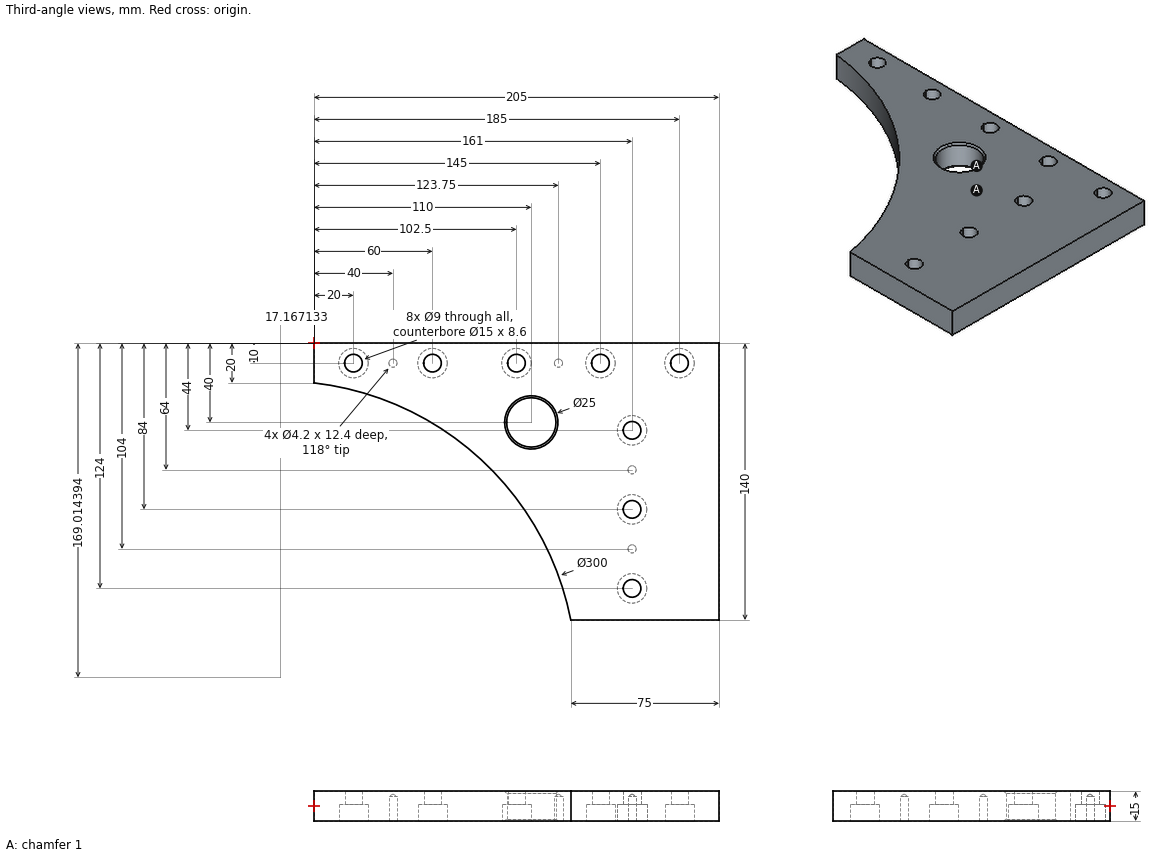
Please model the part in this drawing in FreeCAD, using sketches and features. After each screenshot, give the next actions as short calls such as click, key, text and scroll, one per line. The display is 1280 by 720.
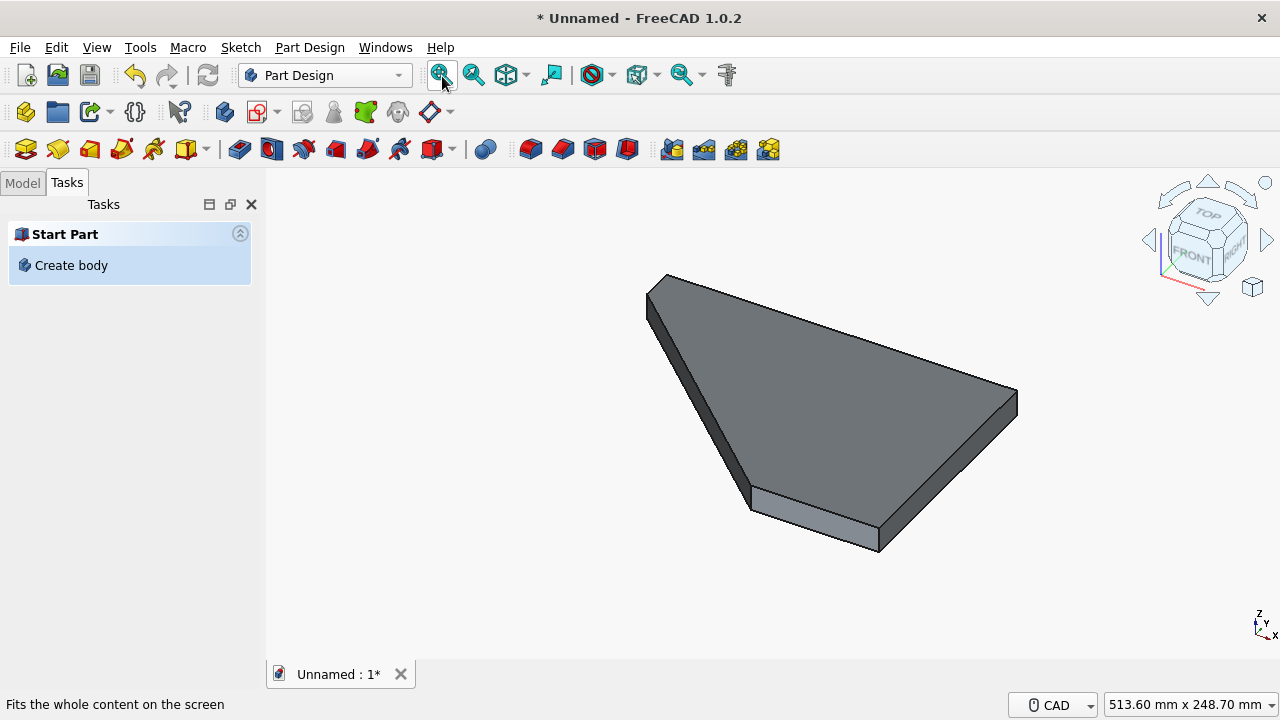
key(5)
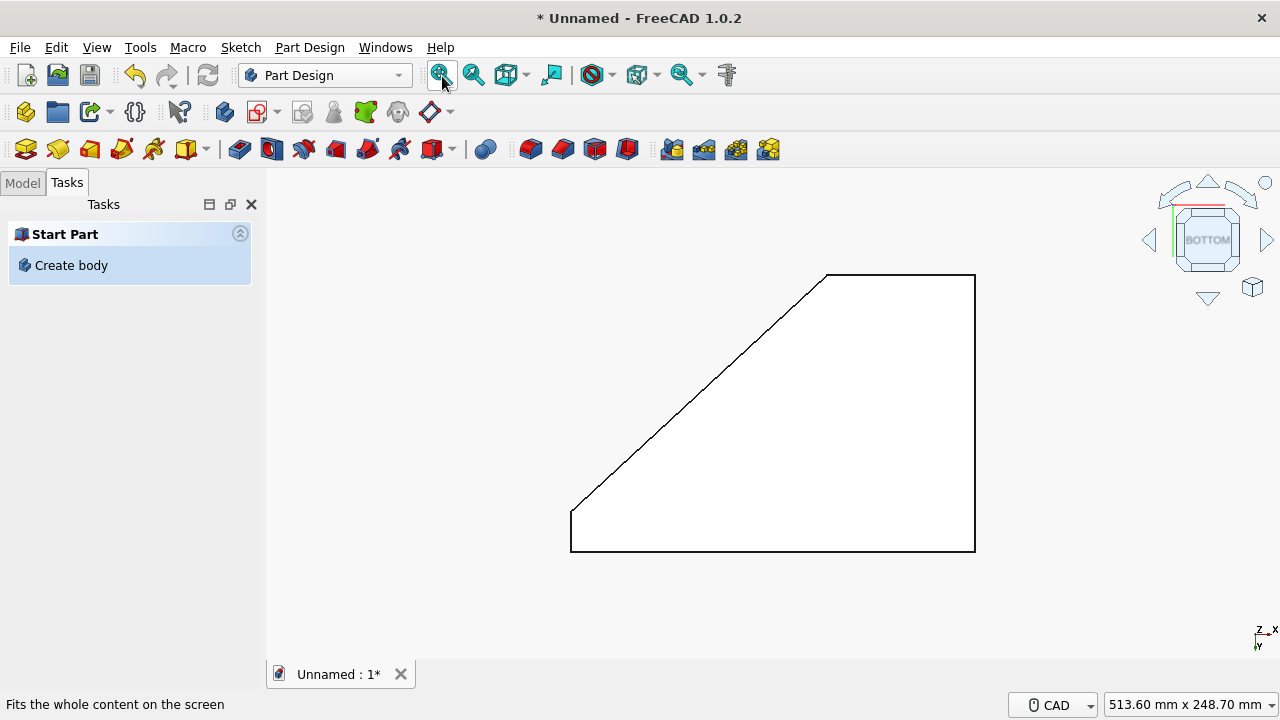
click(831, 412)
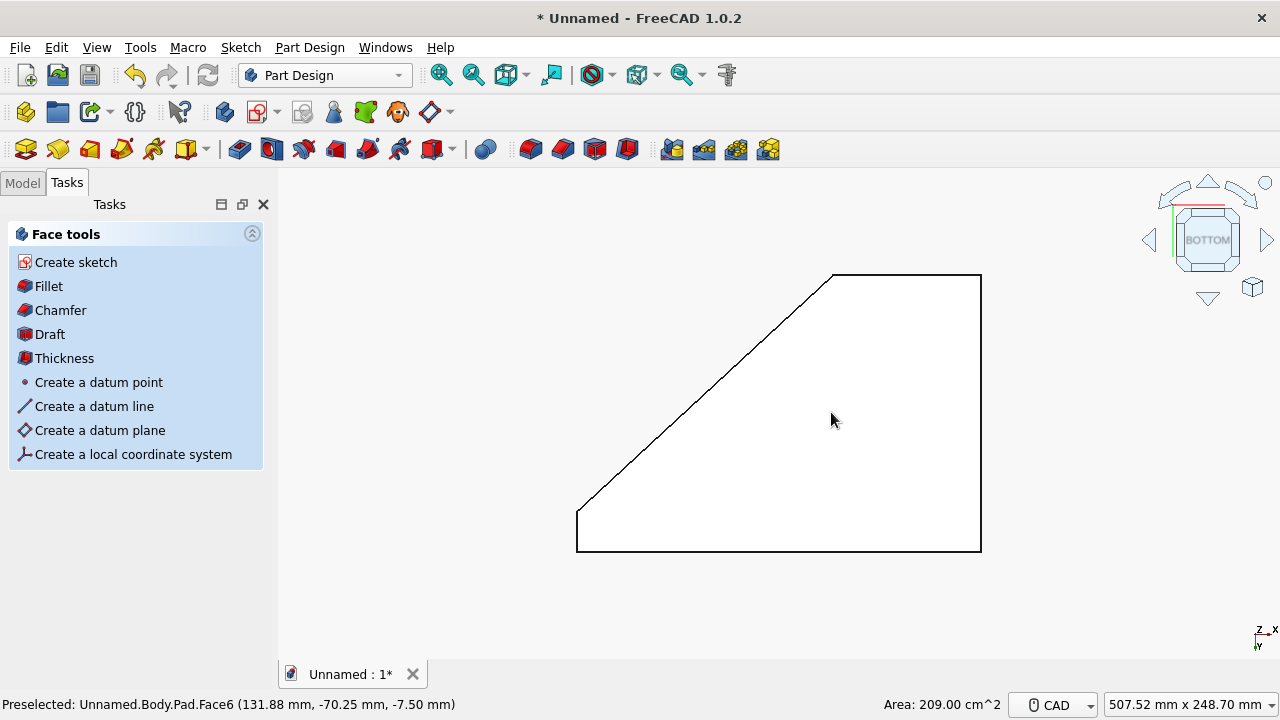
click(258, 112)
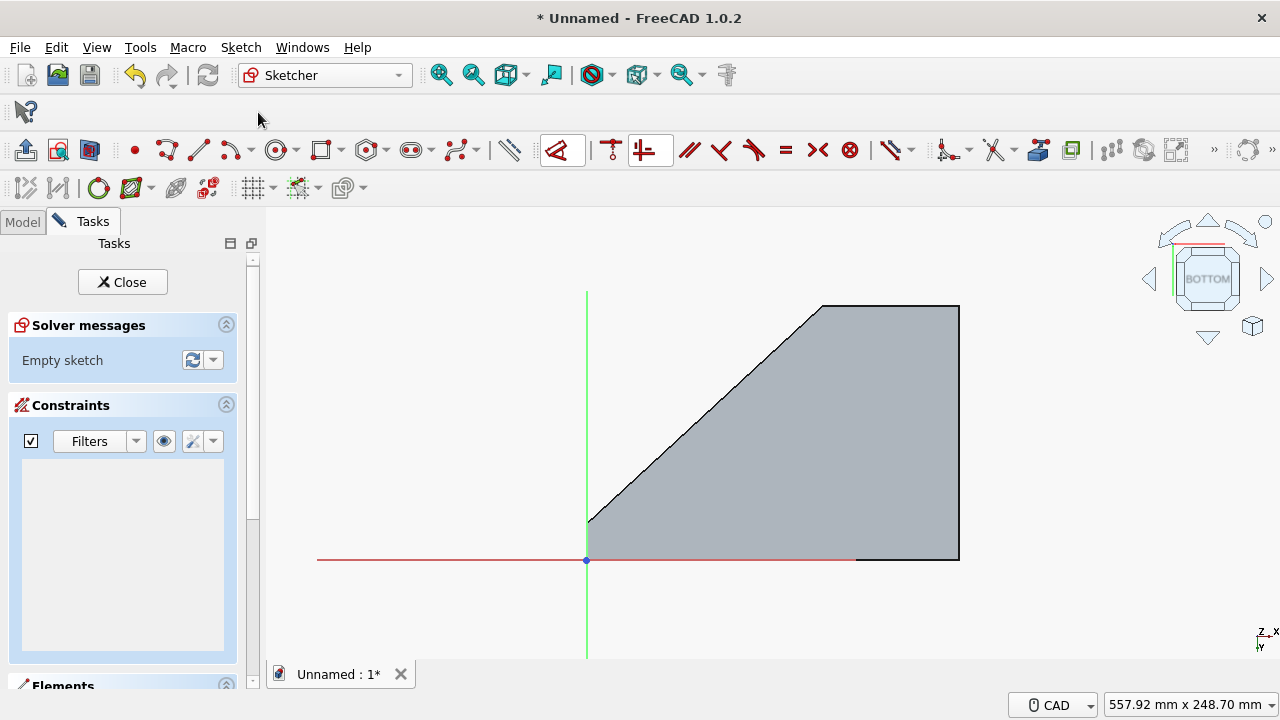
click(276, 150)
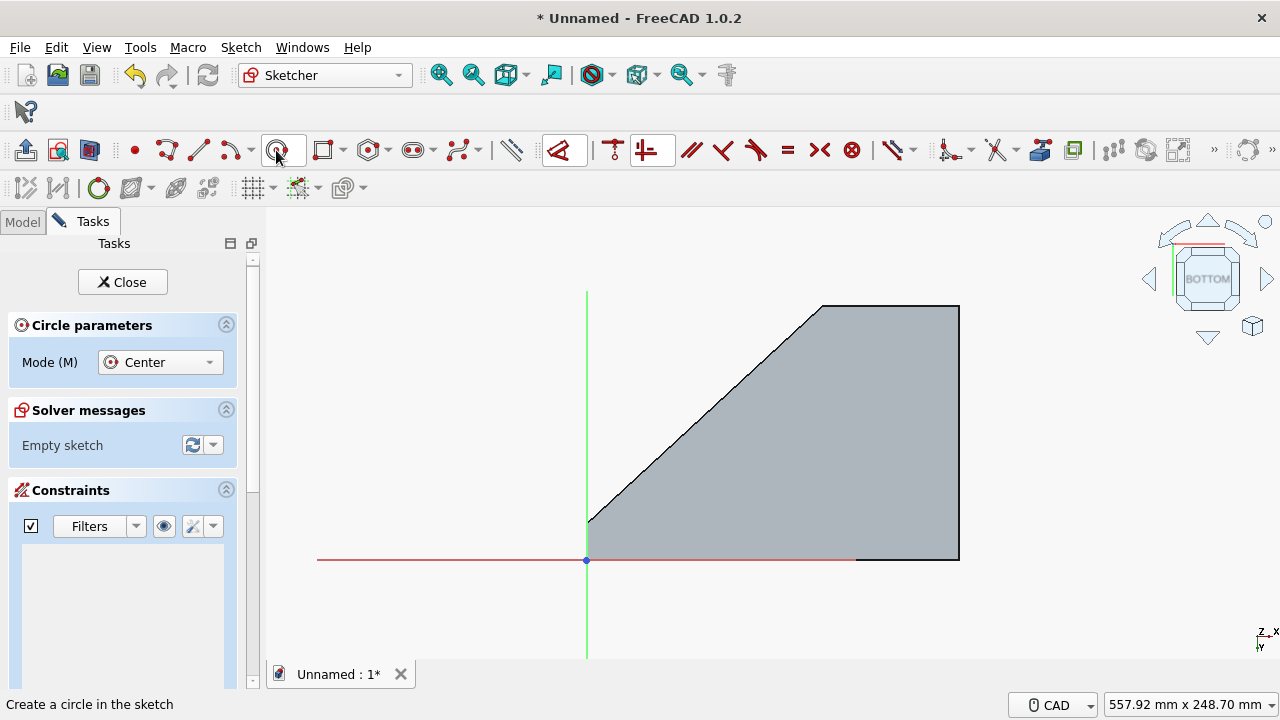
scroll(623, 542, up, 6)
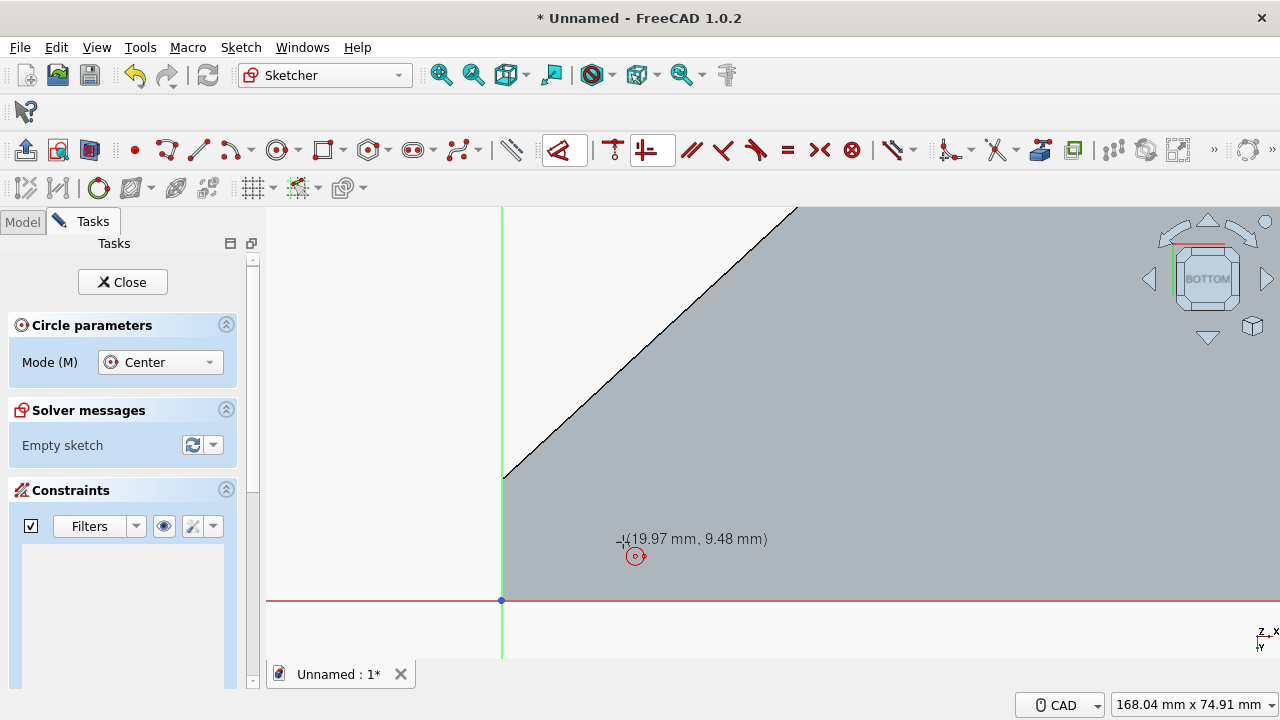
click(622, 540)
click(642, 521)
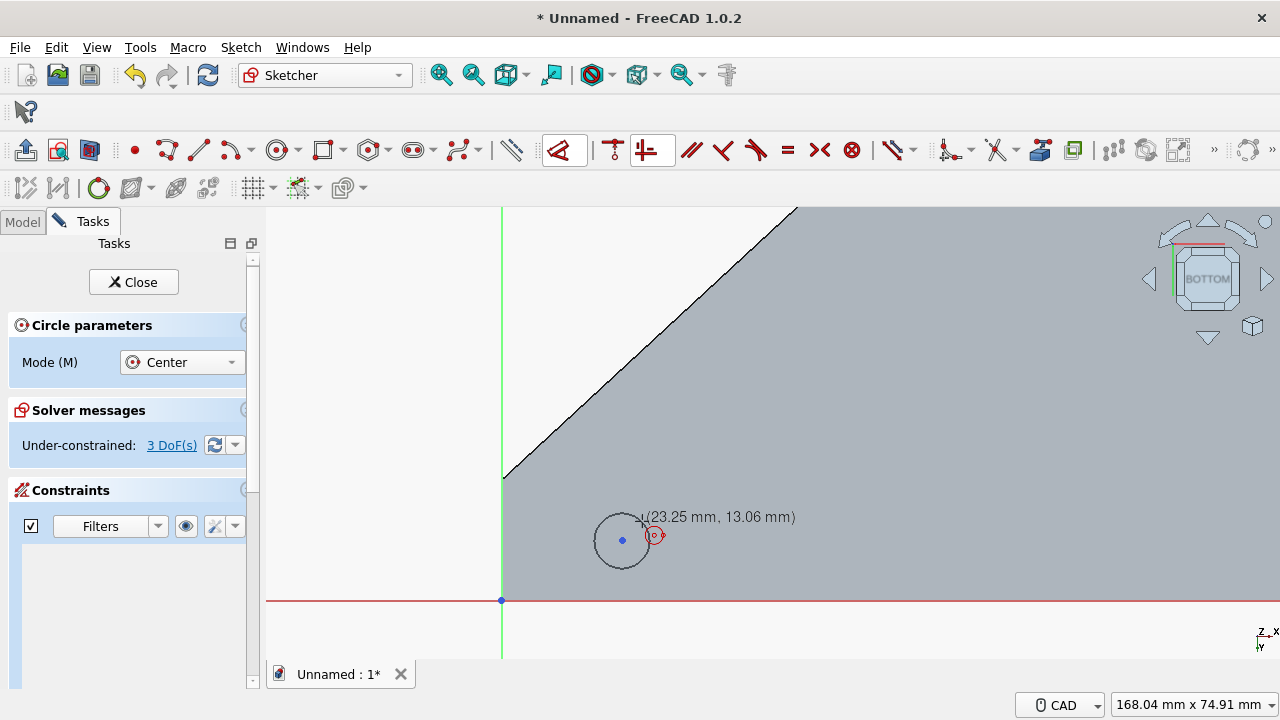
click(864, 540)
click(883, 521)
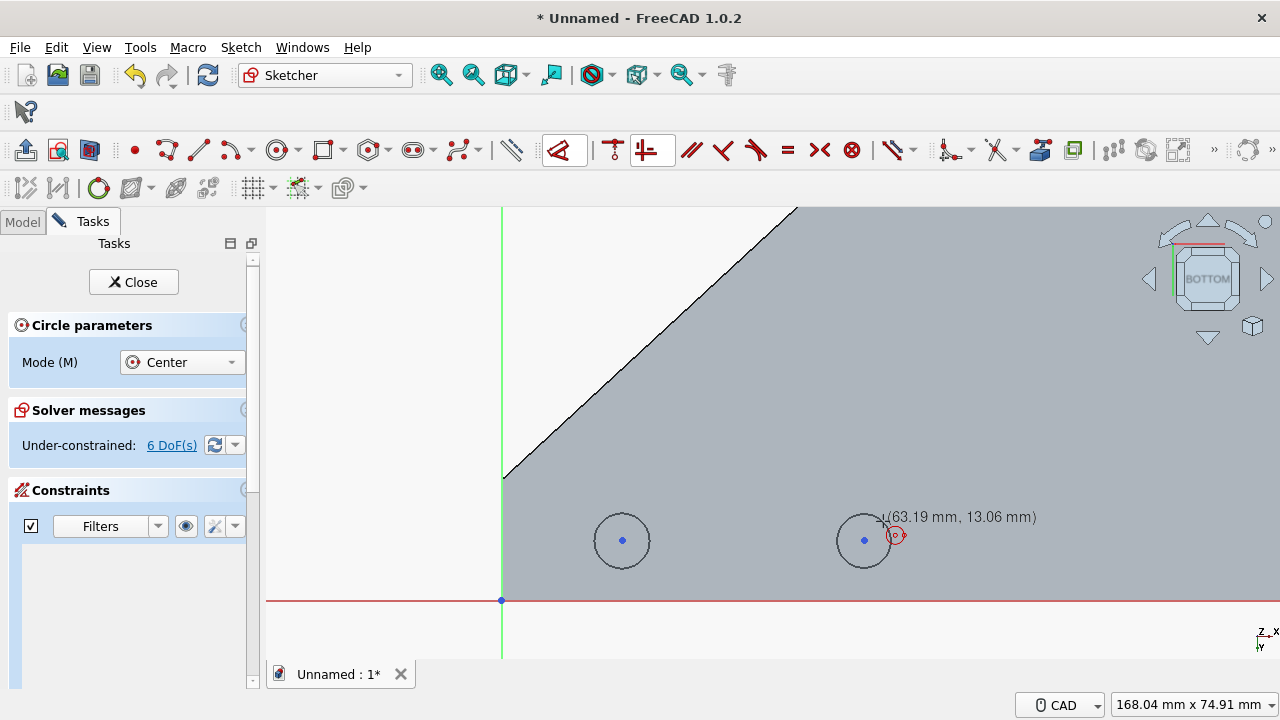
scroll(490, 561, down, 5)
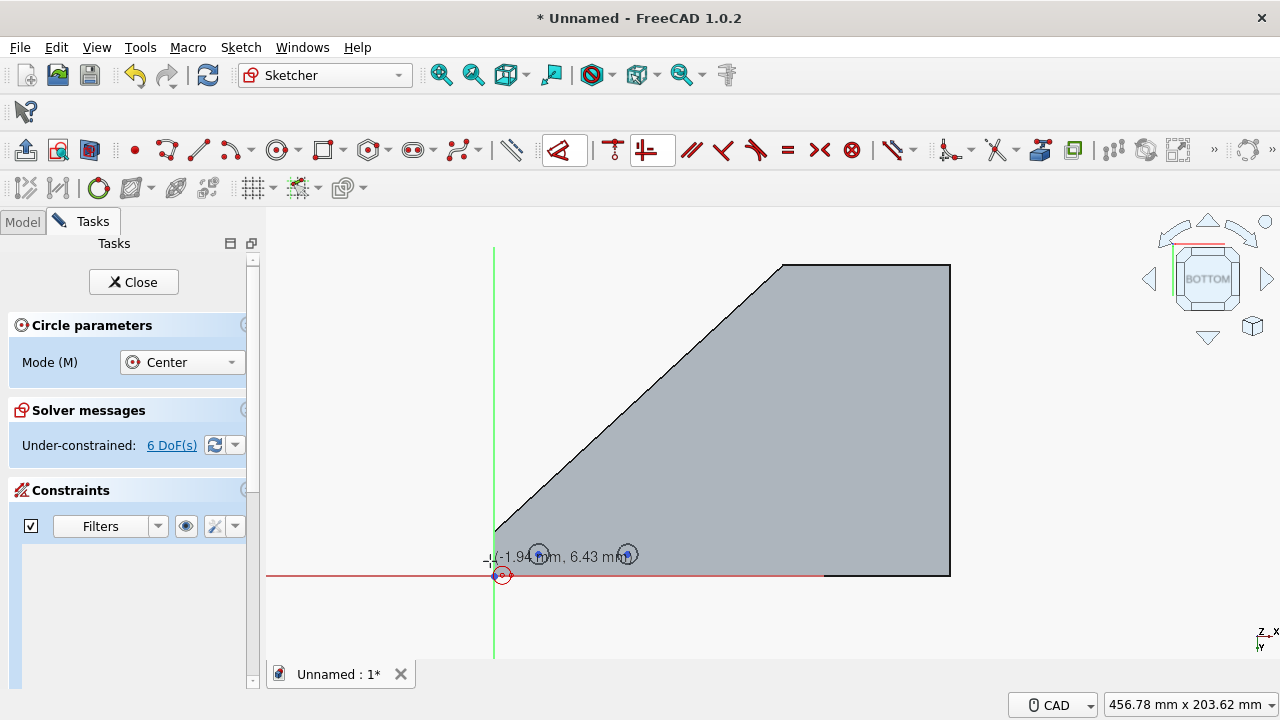
scroll(722, 554, up, 5)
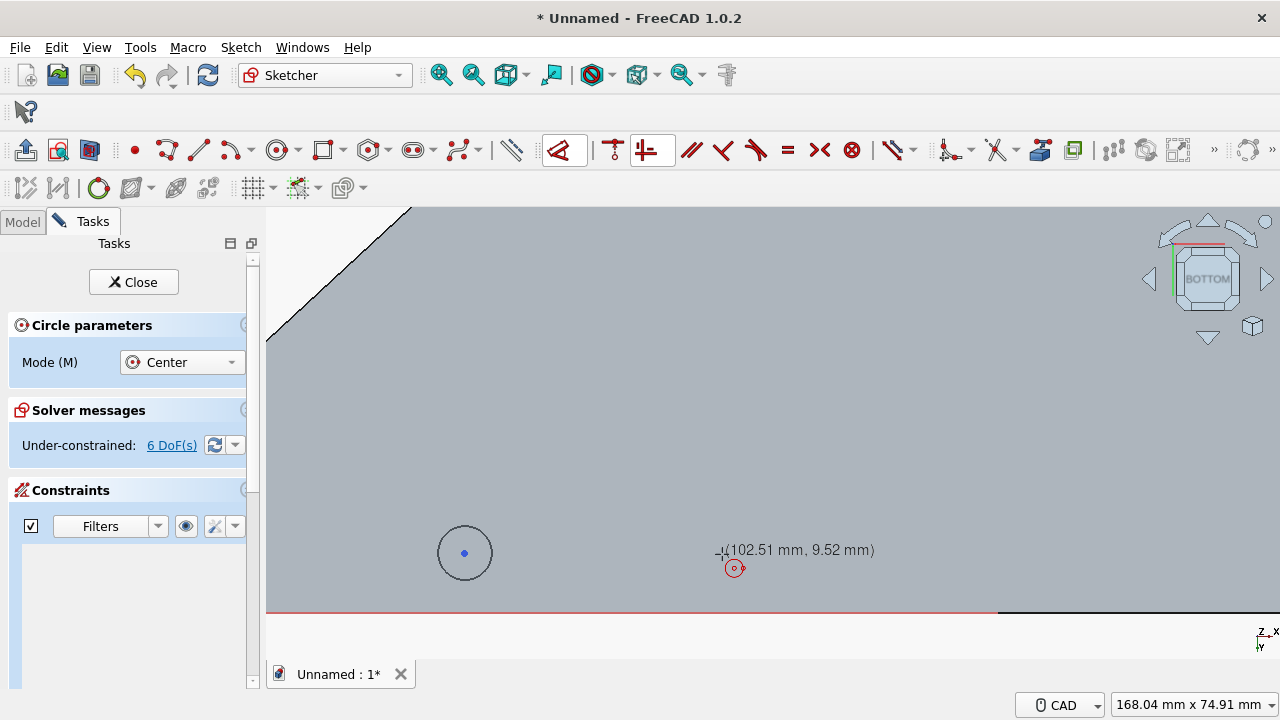
click(721, 552)
click(740, 533)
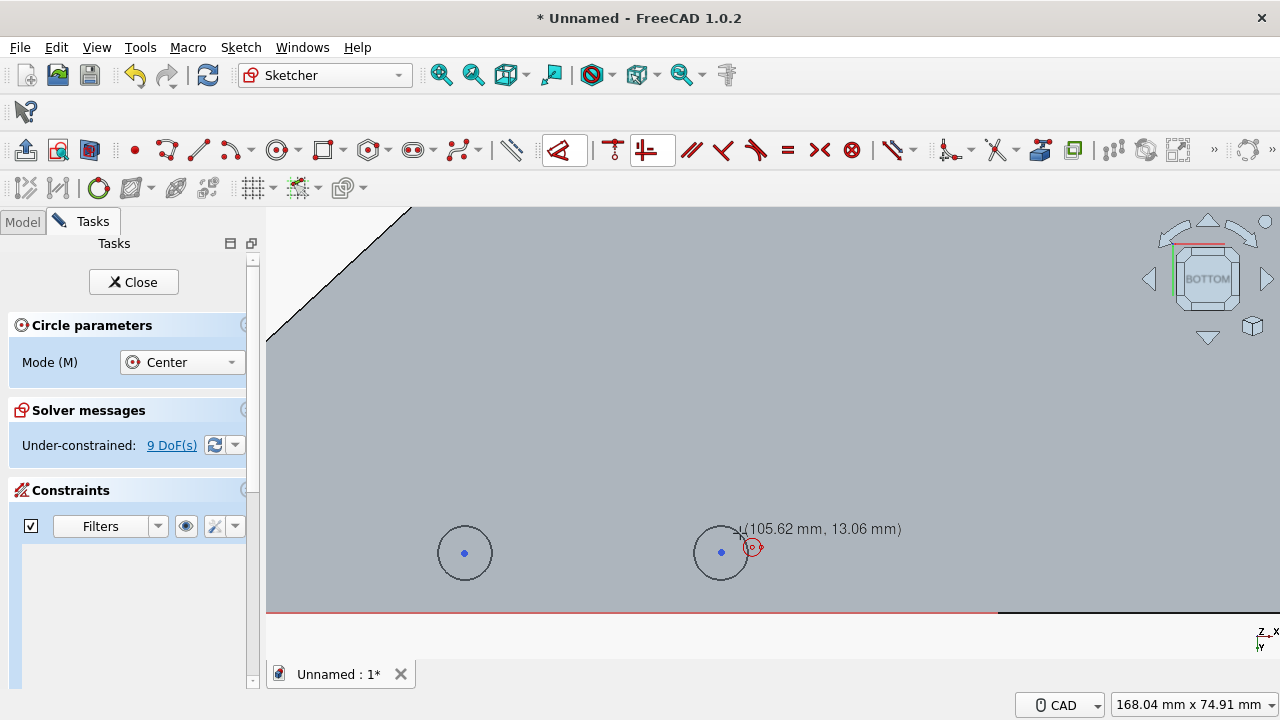
click(978, 552)
click(997, 533)